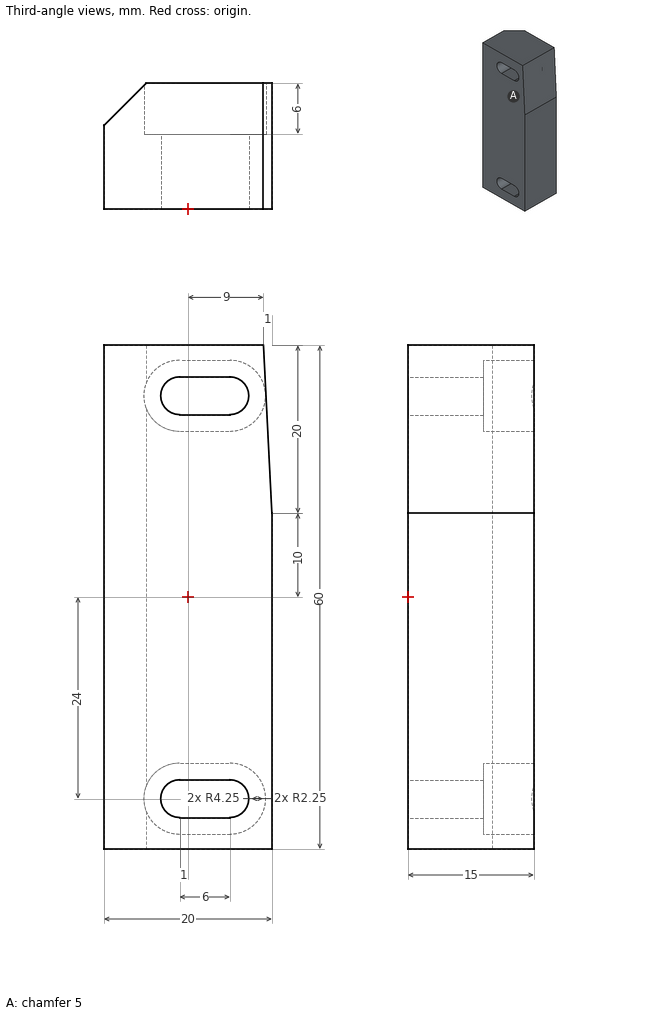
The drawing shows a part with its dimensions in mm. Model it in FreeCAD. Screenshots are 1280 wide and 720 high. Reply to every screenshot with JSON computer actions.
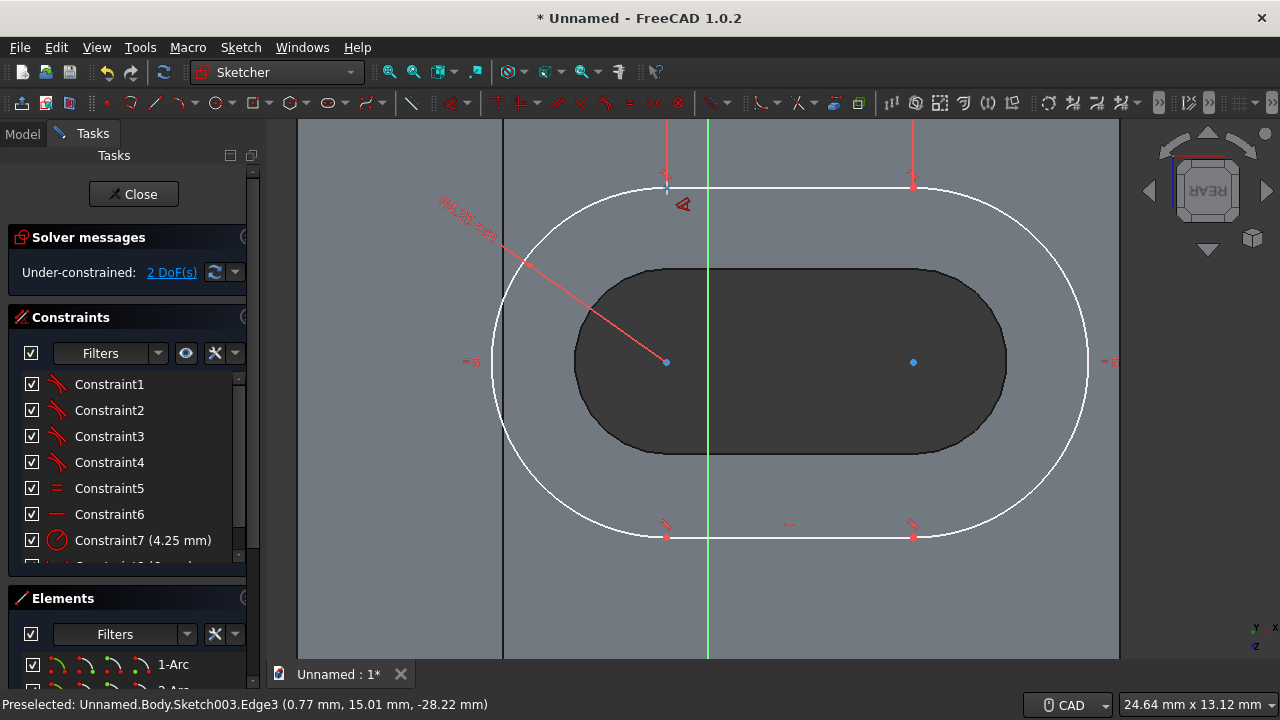
{"action": "left_click", "coordinate": [667, 188]}
{"action": "left_click", "coordinate": [687, 154]}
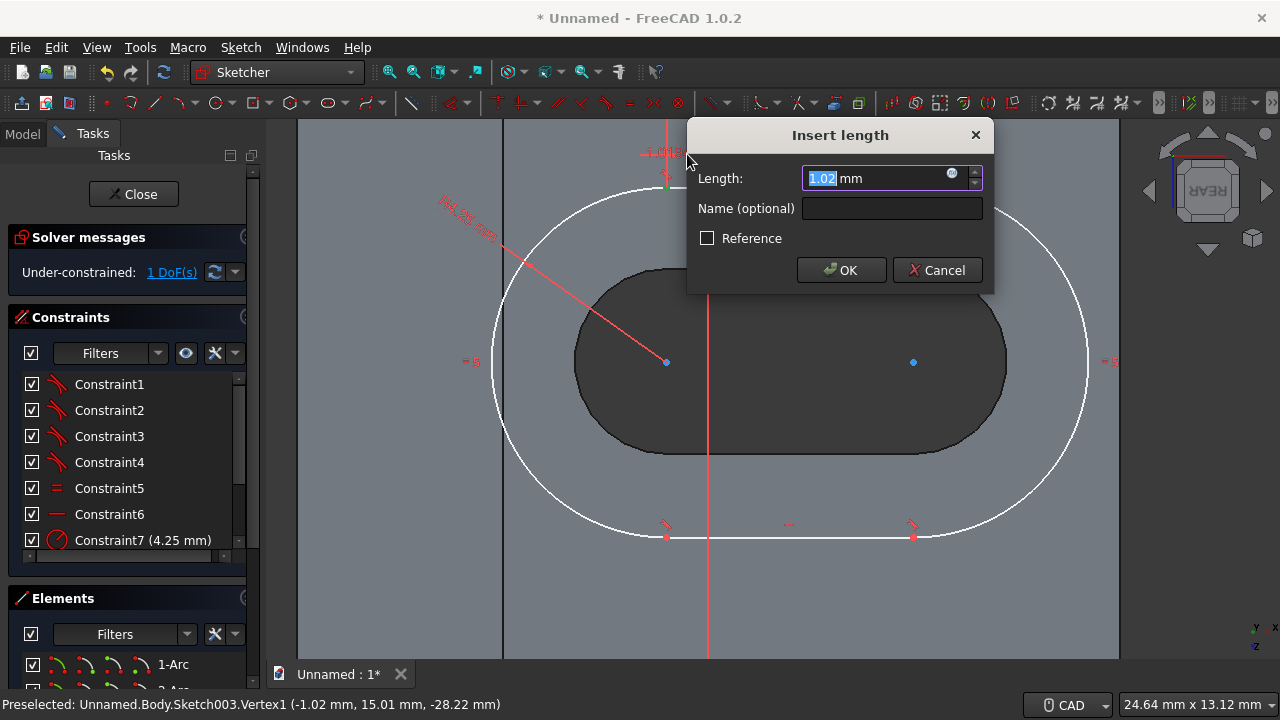
{"action": "type", "text": "1"}
{"action": "key", "text": "Return"}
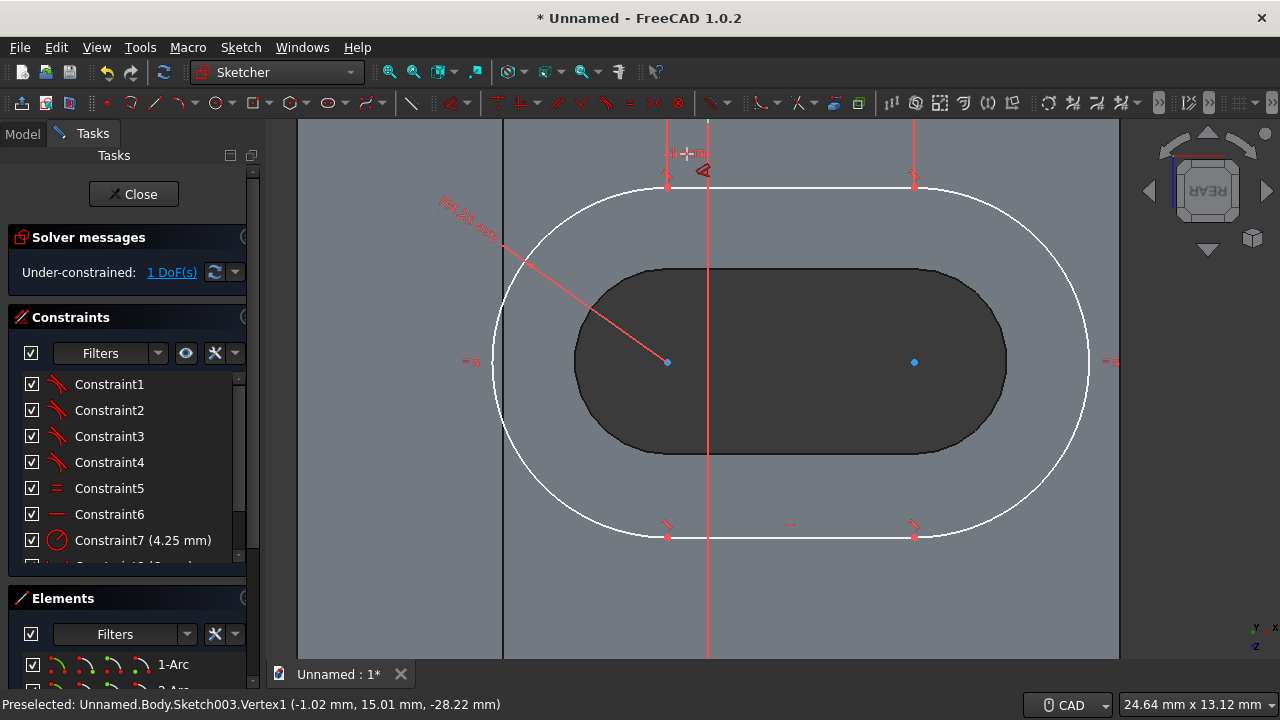
{"action": "left_click", "coordinate": [667, 363]}
{"action": "left_click", "coordinate": [633, 497]}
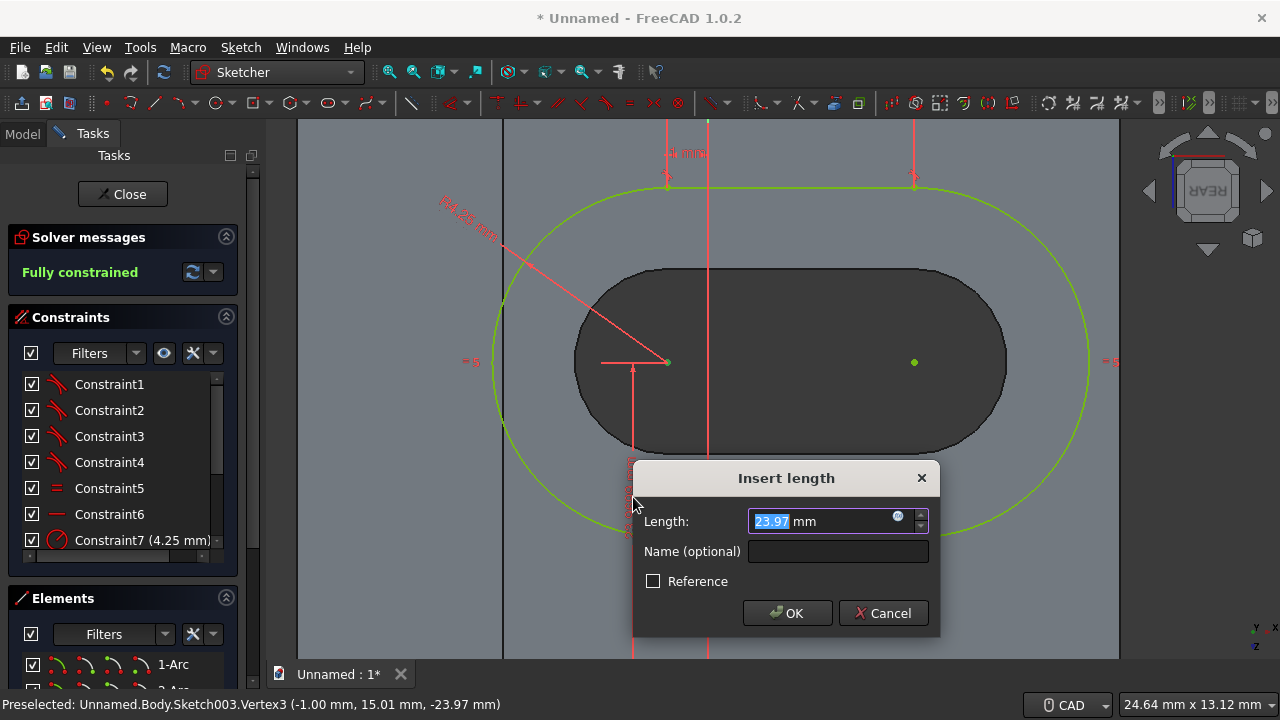
{"action": "type", "text": "24"}
{"action": "key", "text": "Return"}
{"action": "key", "text": "Escape"}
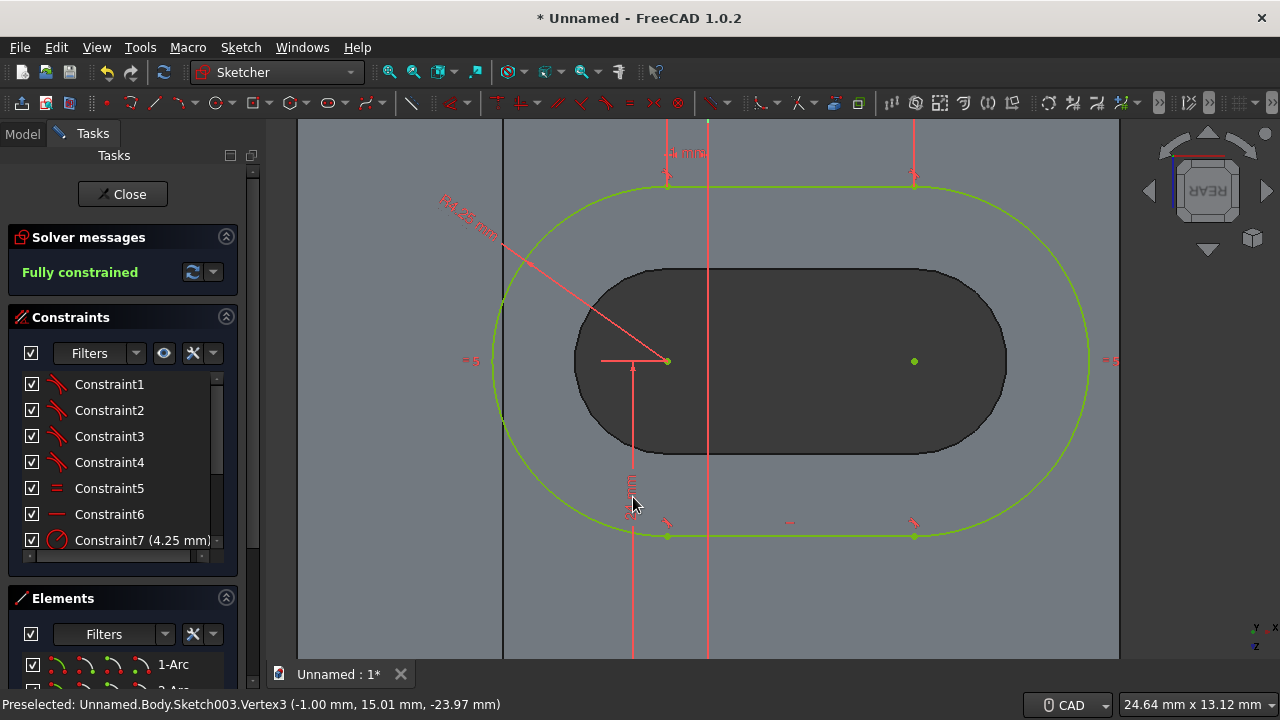
{"action": "left_click", "coordinate": [123, 194]}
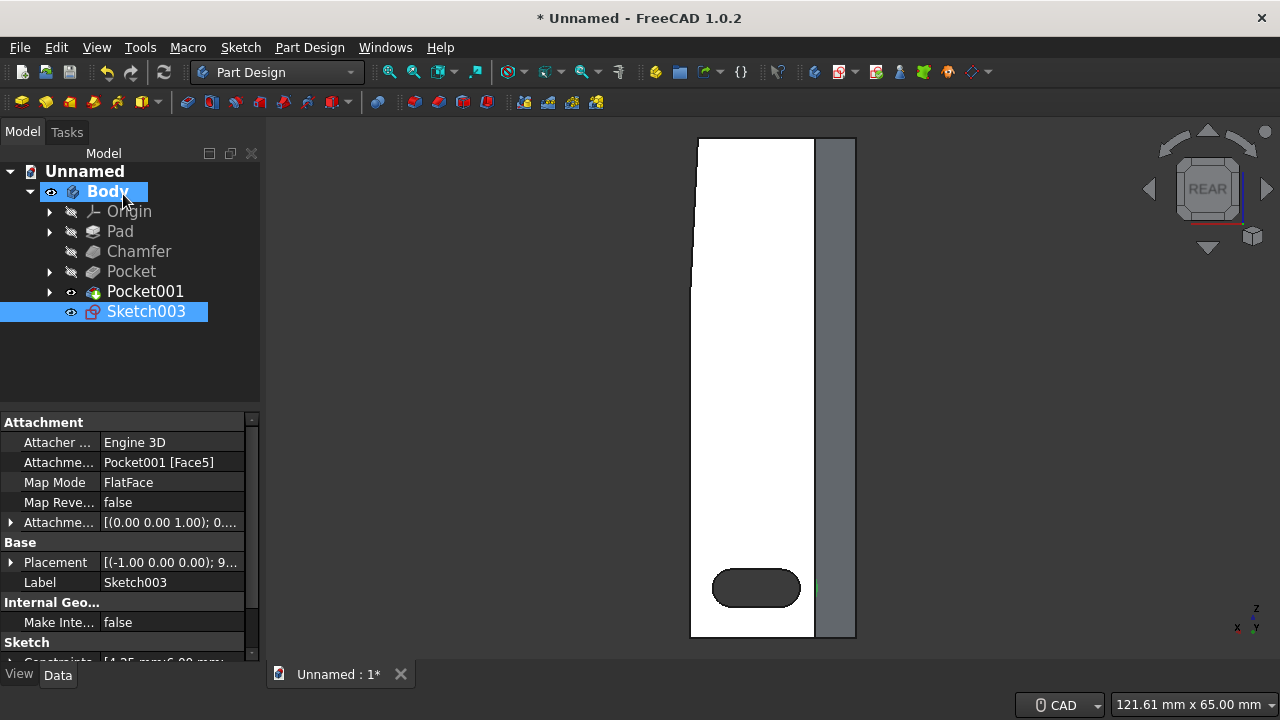
{"action": "left_click", "coordinate": [188, 102]}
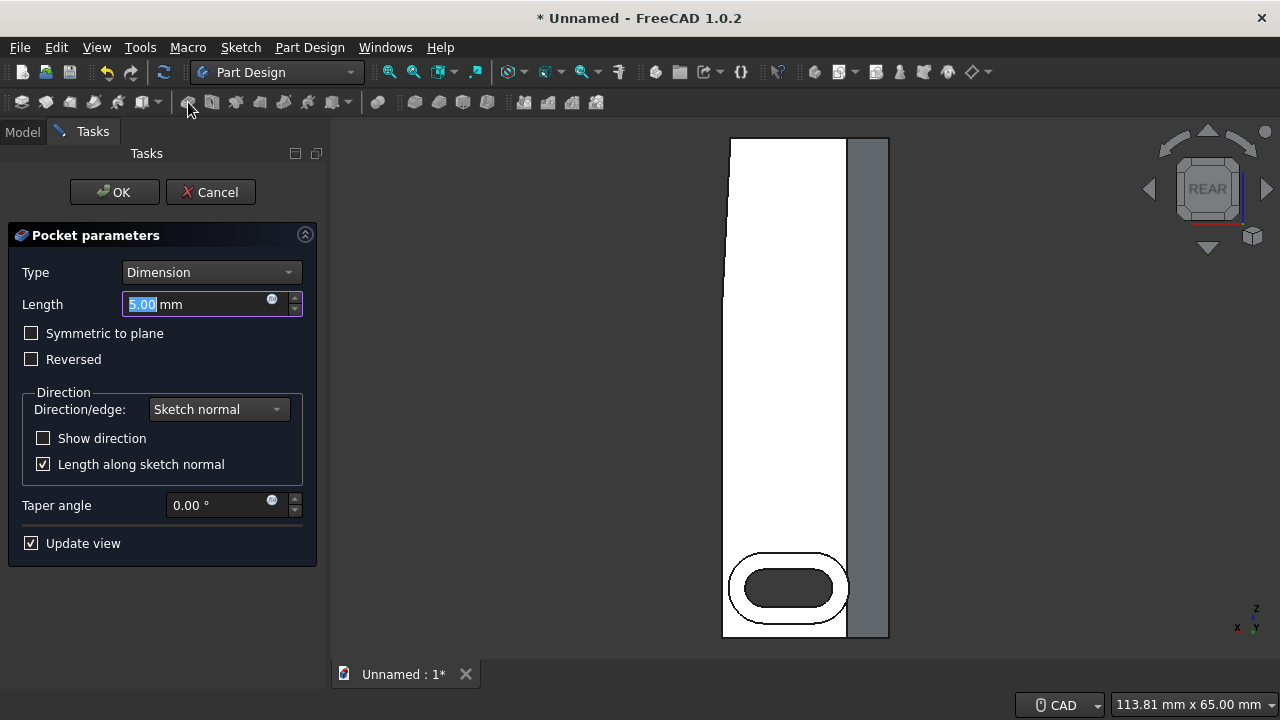
{"action": "type", "text": "6"}
{"action": "key", "text": "Tab"}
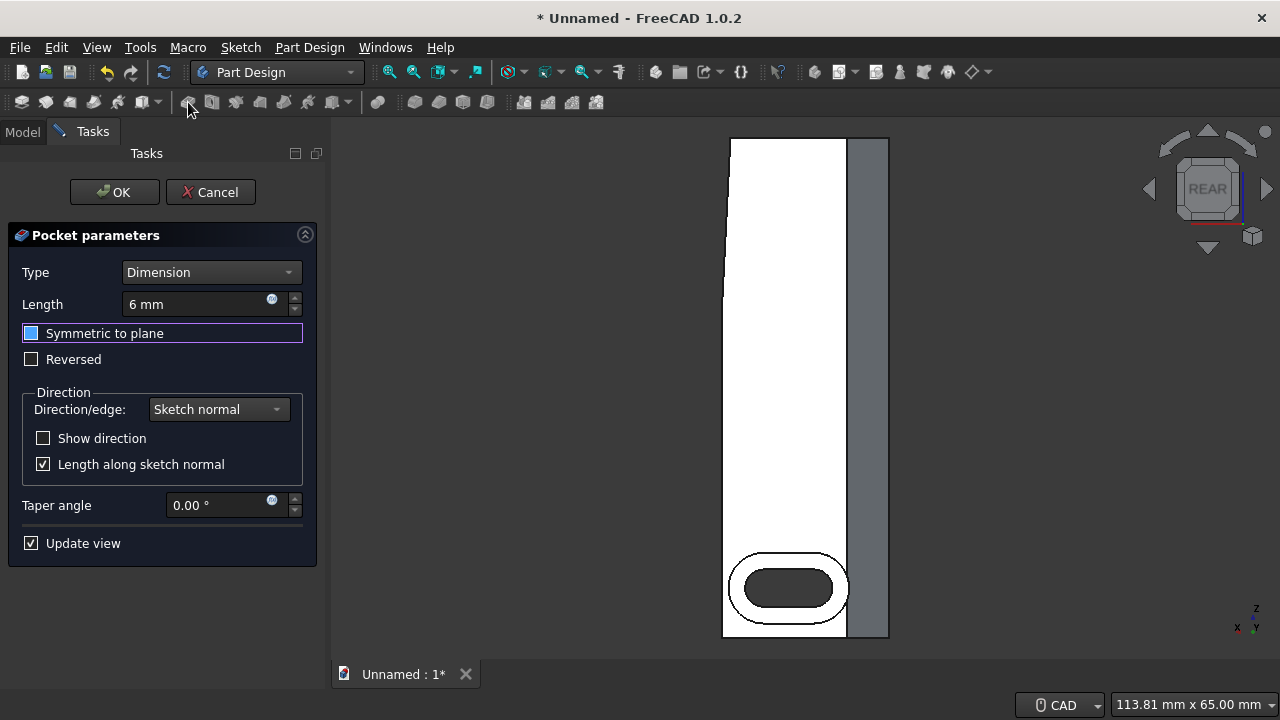
{"action": "left_click", "coordinate": [115, 192]}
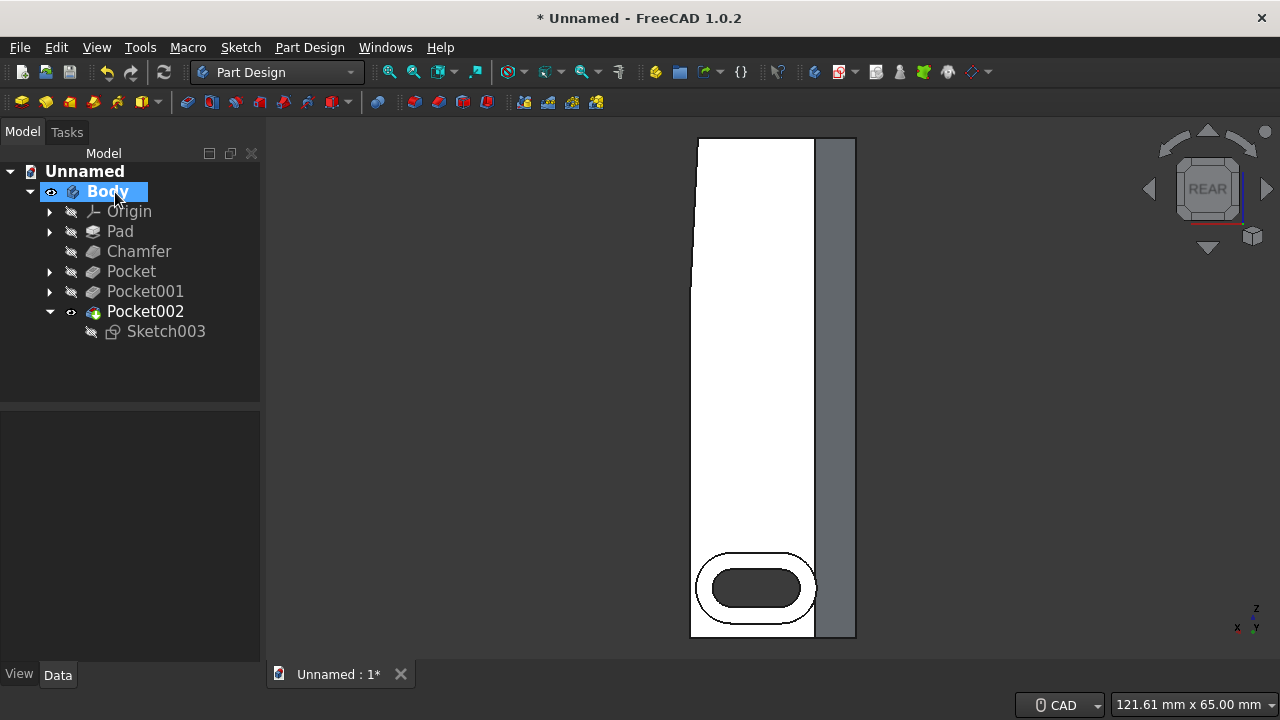
{"action": "left_click", "coordinate": [116, 292]}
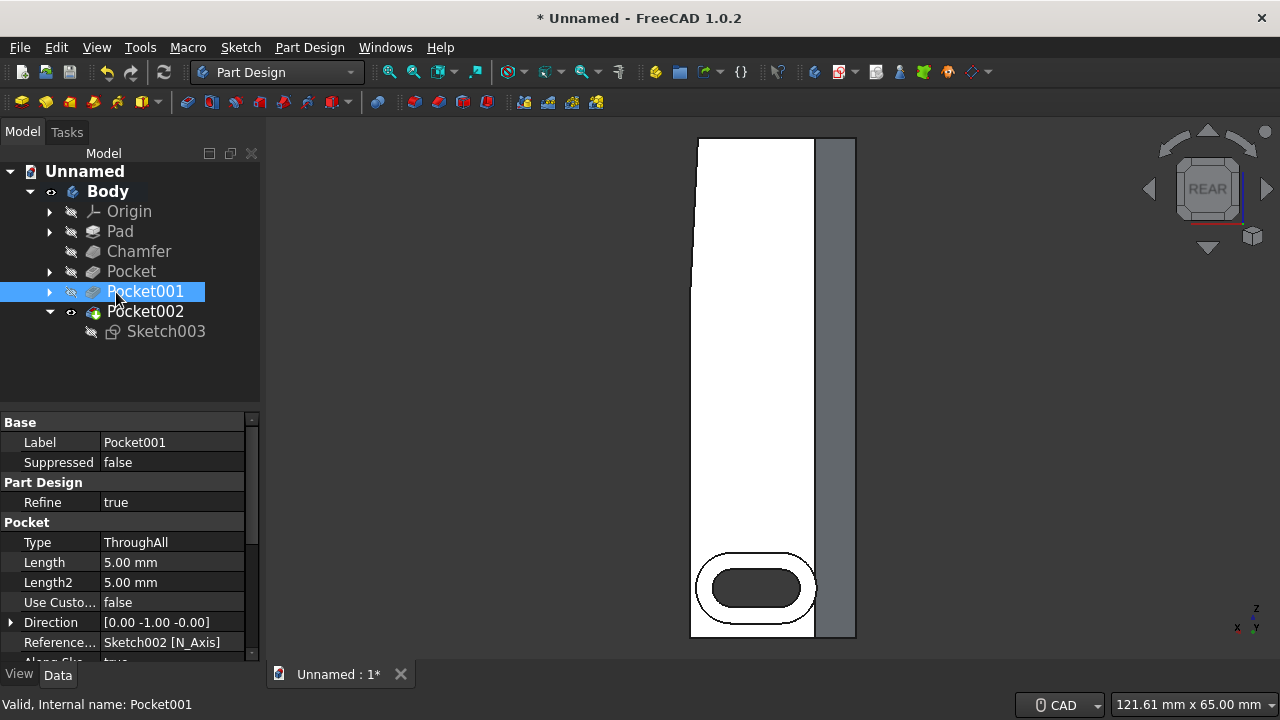
{"action": "left_click", "coordinate": [116, 312], "text": "ctrl"}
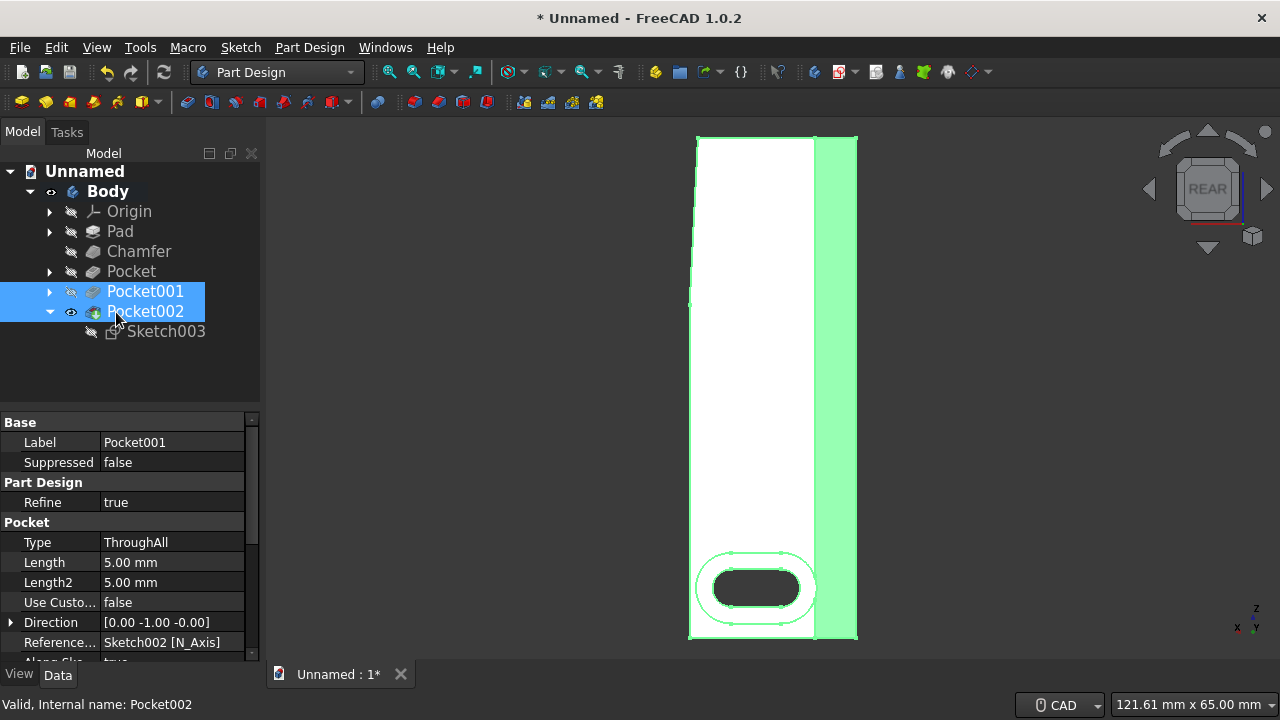
{"action": "left_click", "coordinate": [524, 102]}